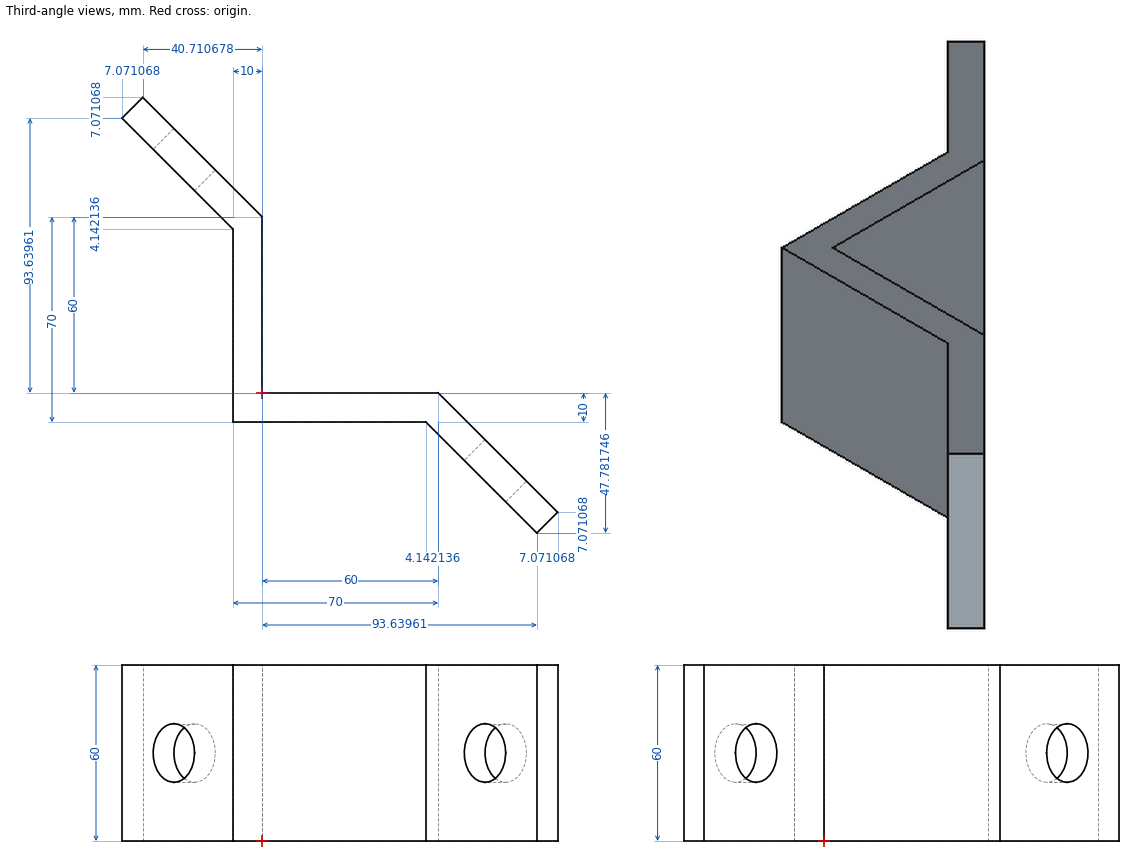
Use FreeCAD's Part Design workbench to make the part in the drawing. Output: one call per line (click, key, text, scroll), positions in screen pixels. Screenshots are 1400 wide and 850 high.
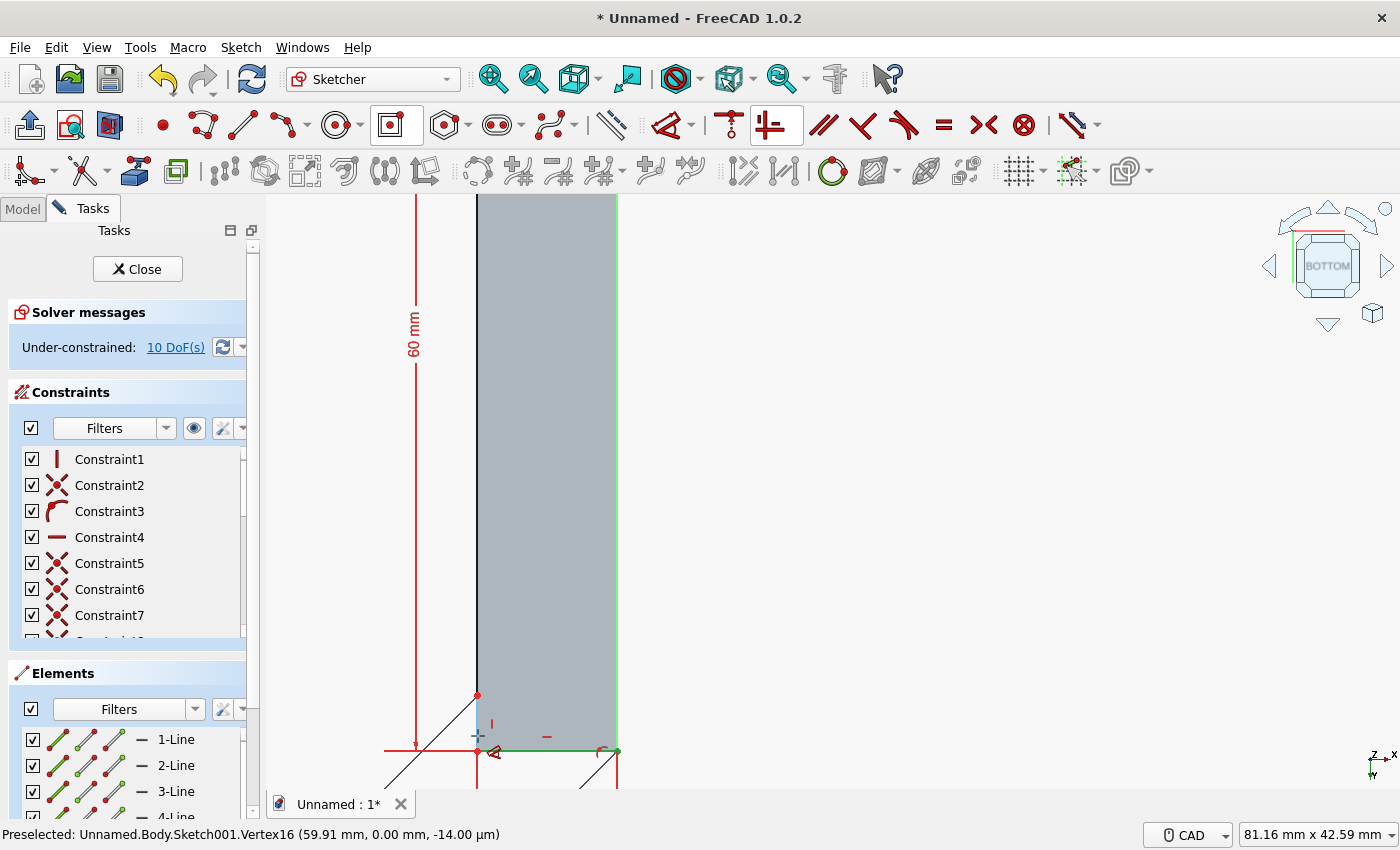
click(477, 735)
click(443, 711)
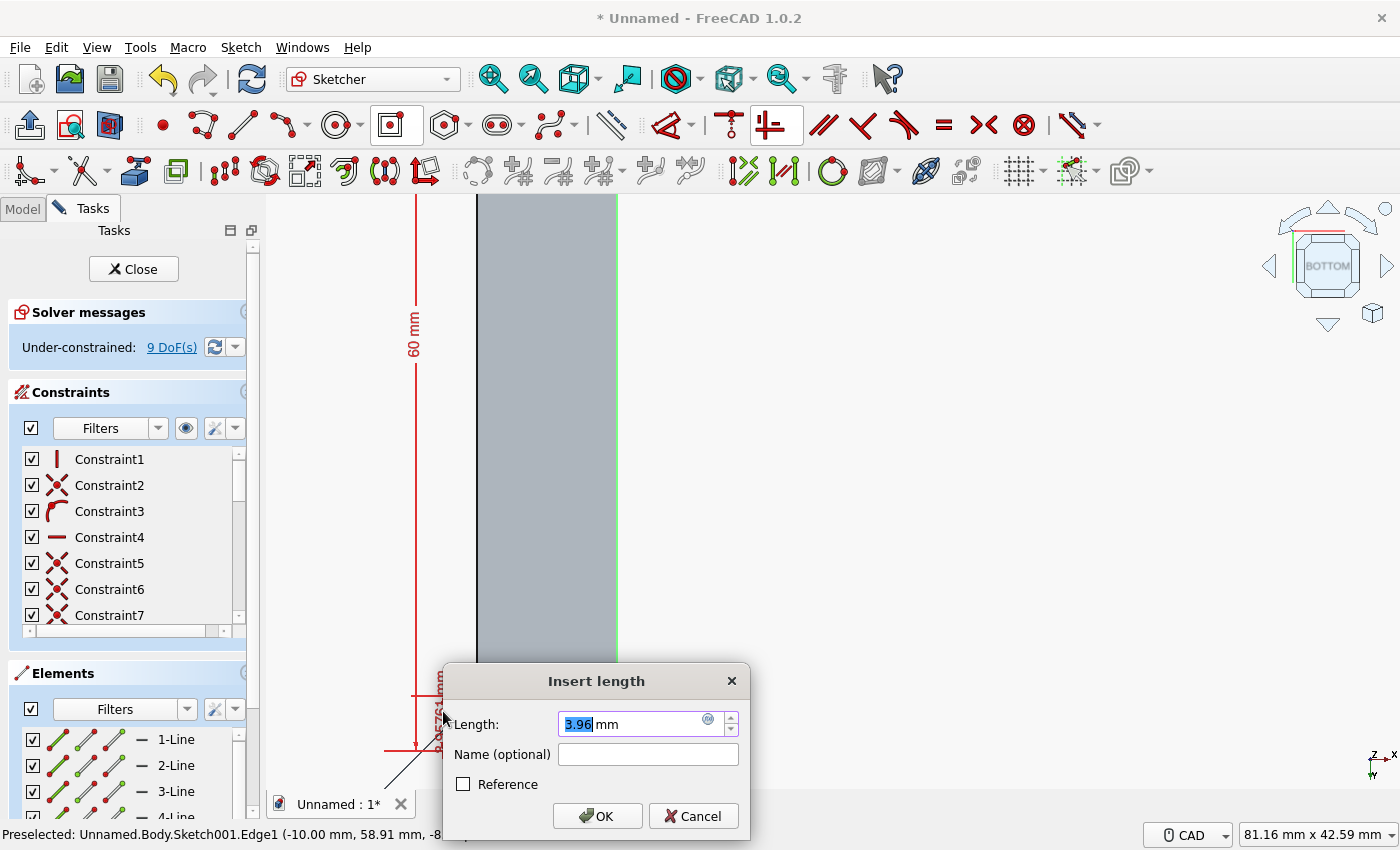
text(4.142136)
key(Return)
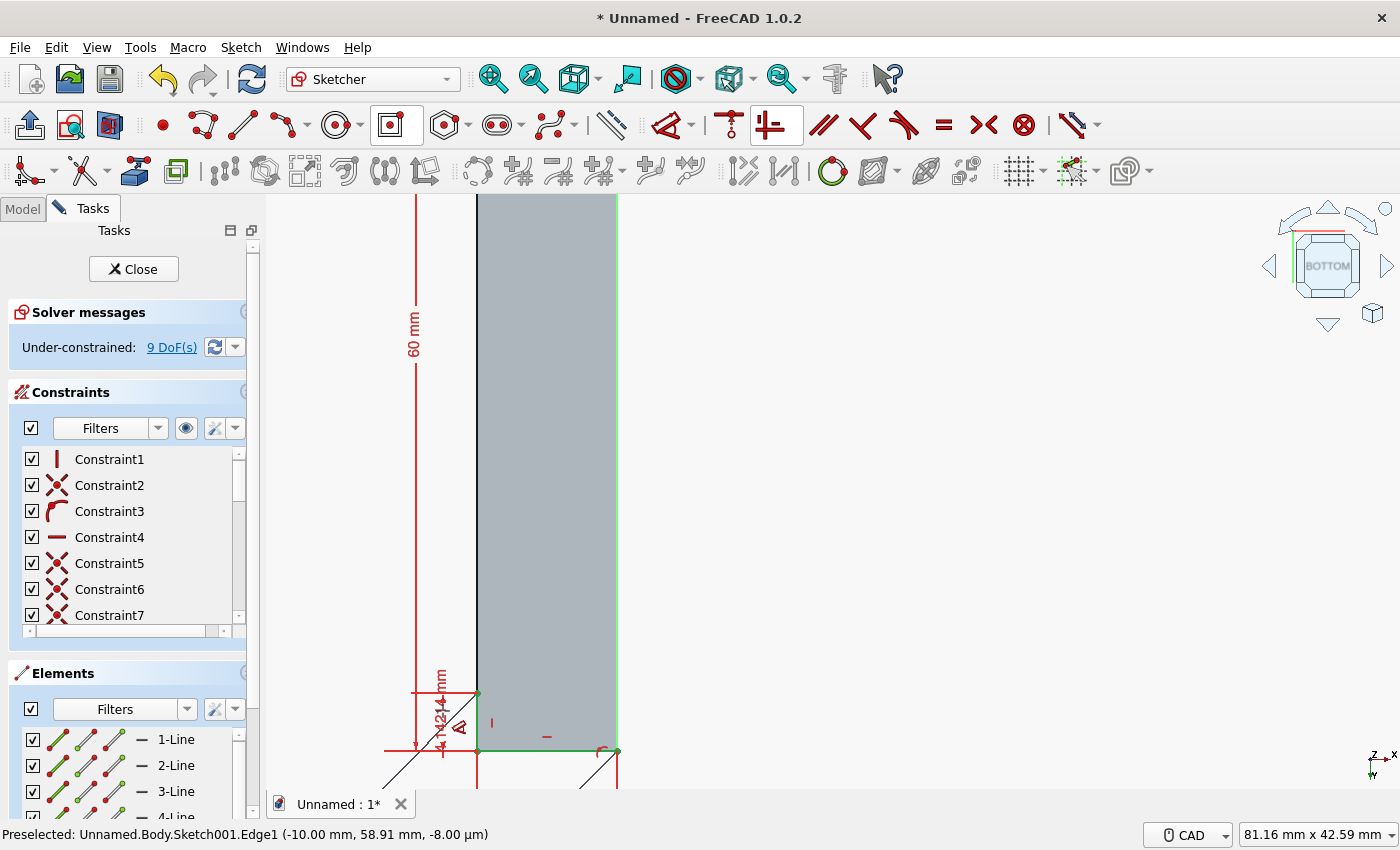
scroll(708, 544, down, 8)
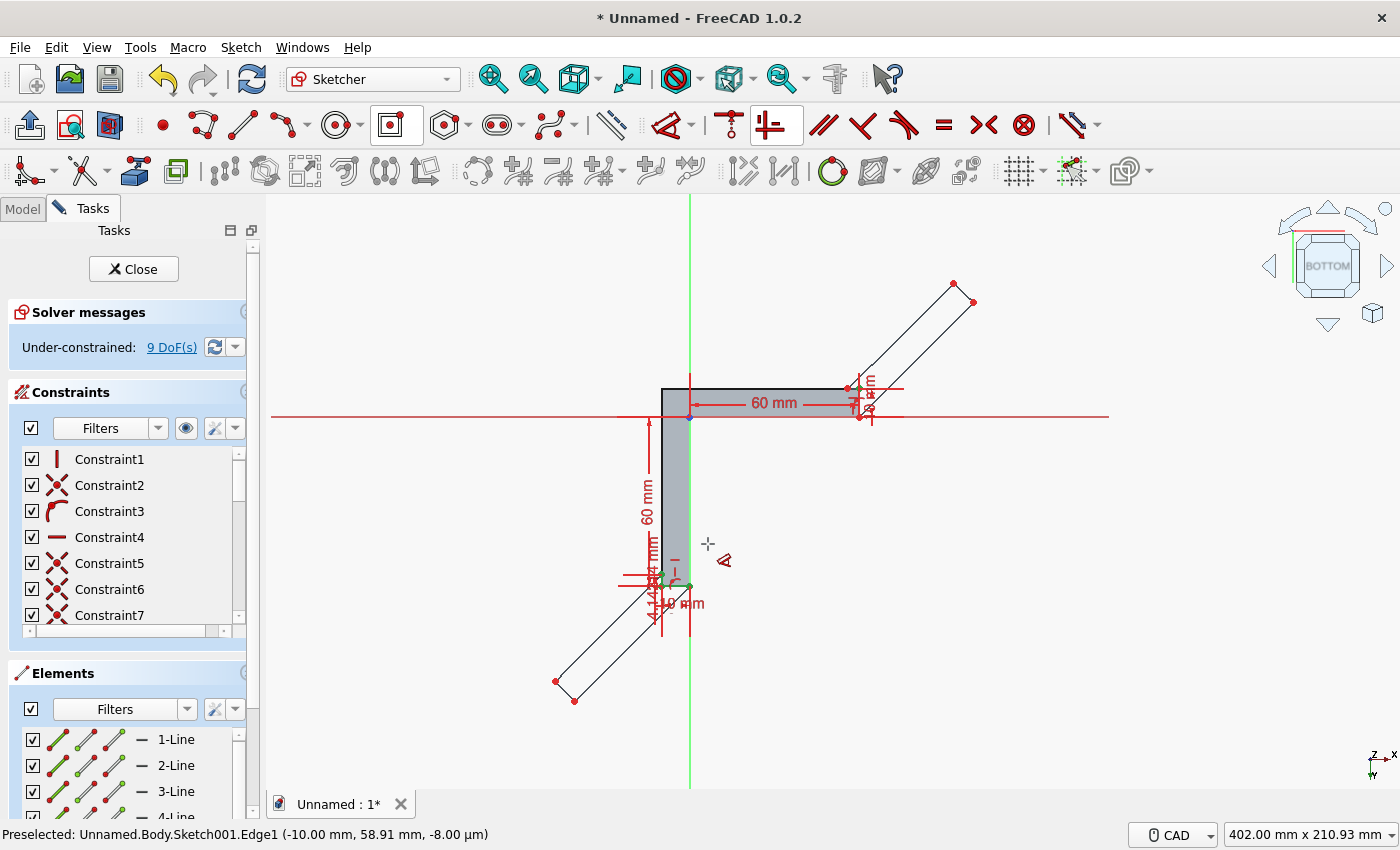
scroll(856, 389, up, 8)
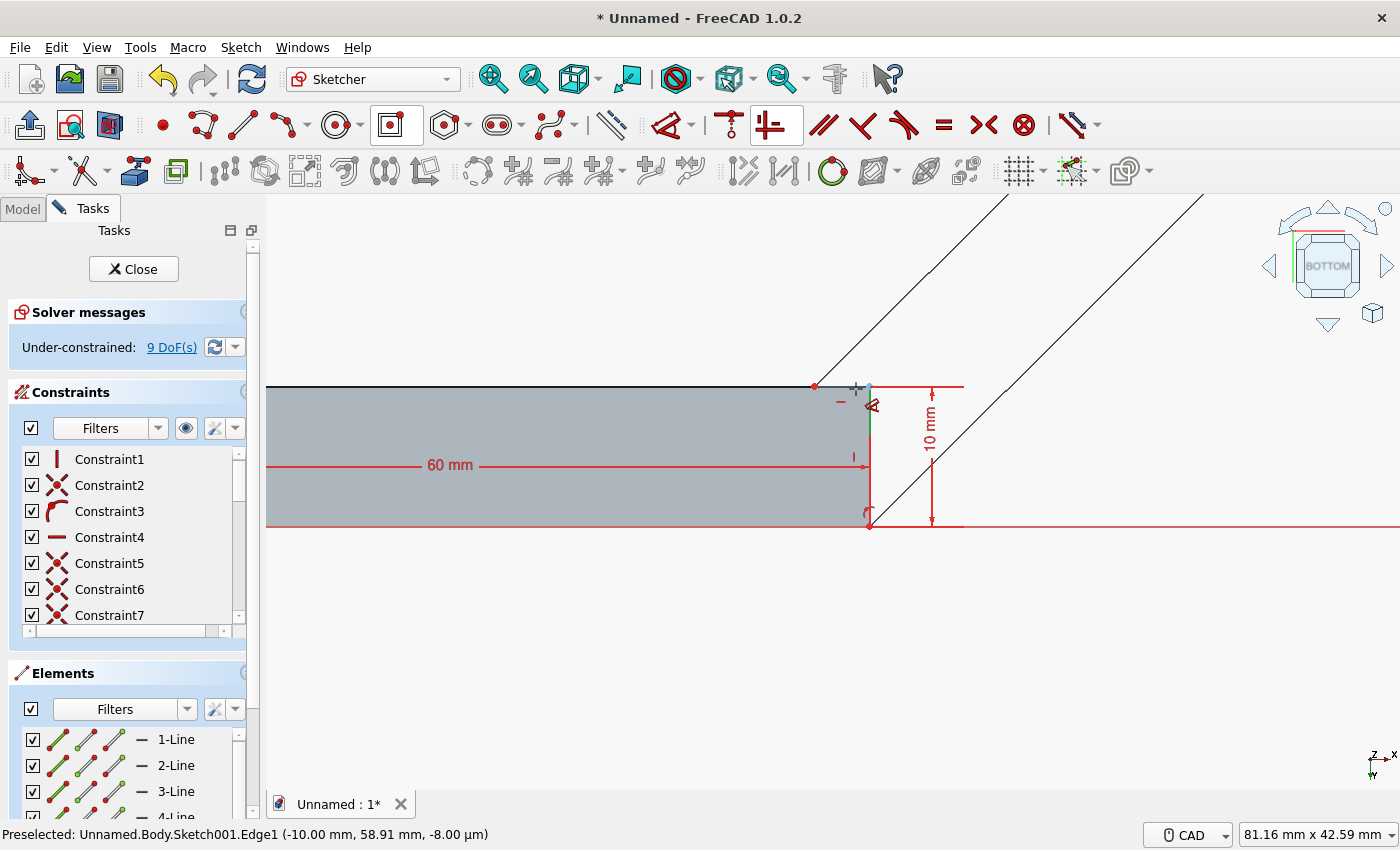
click(853, 387)
click(829, 353)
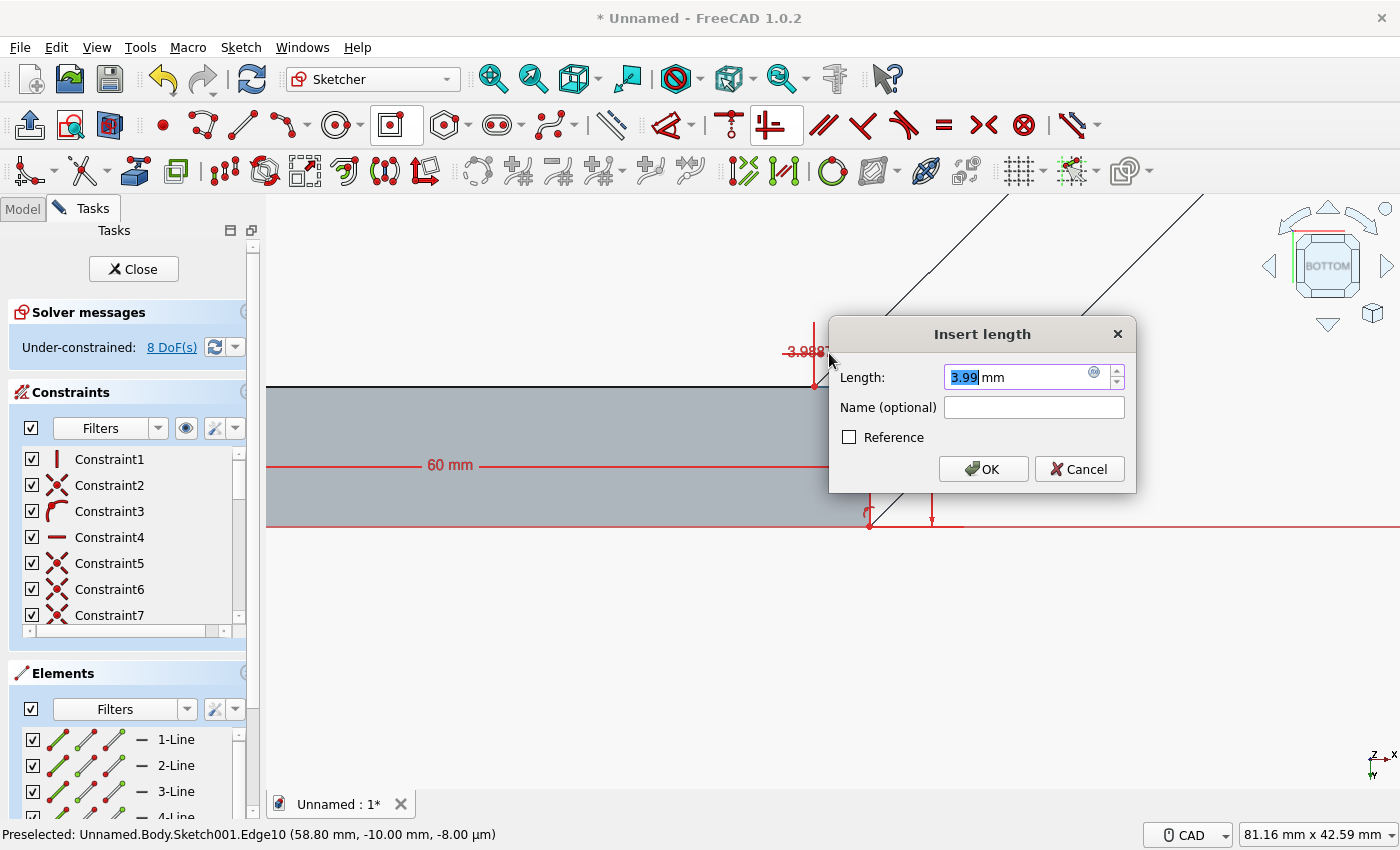
text(4.142136)
key(Return)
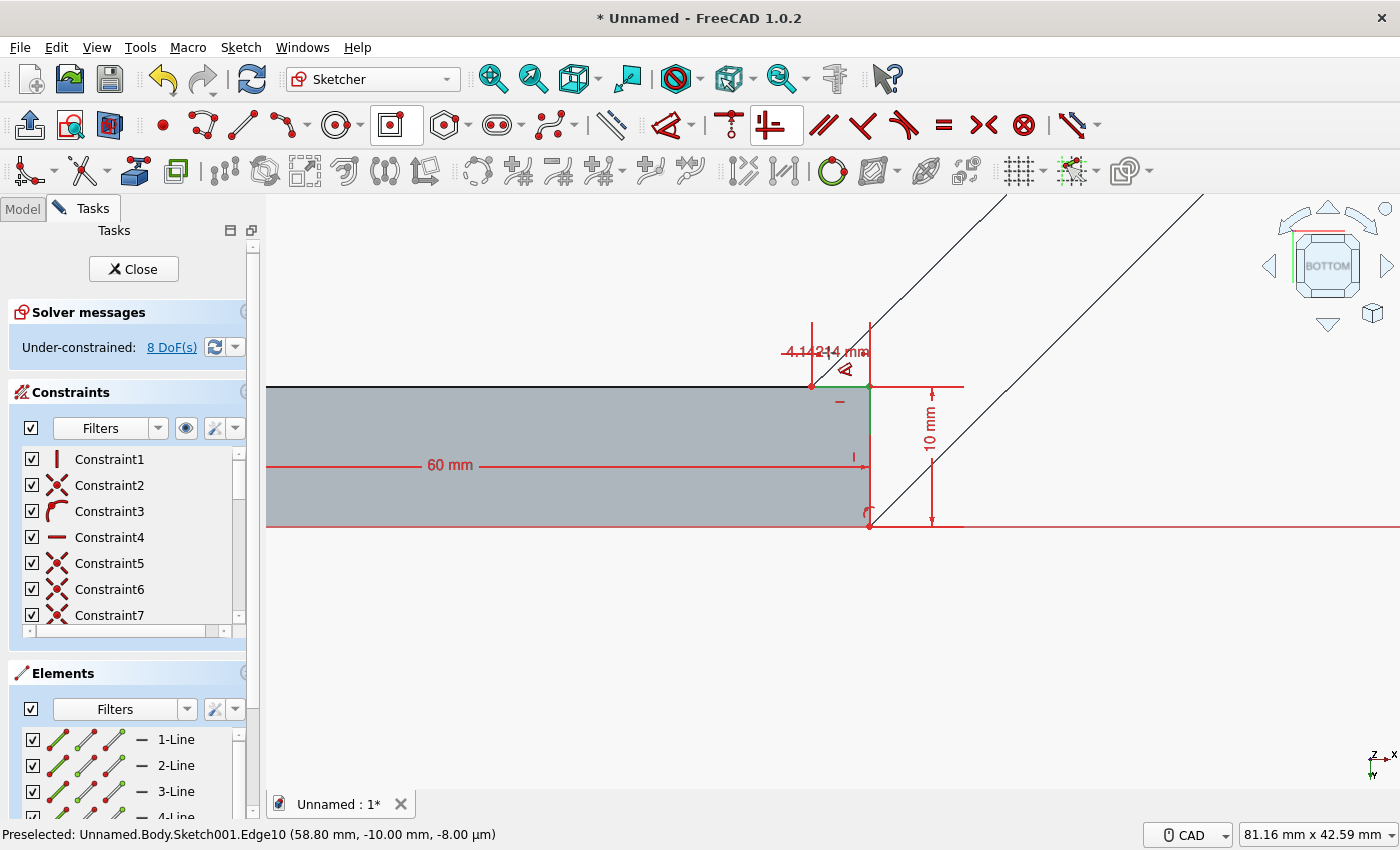
scroll(856, 389, down, 8)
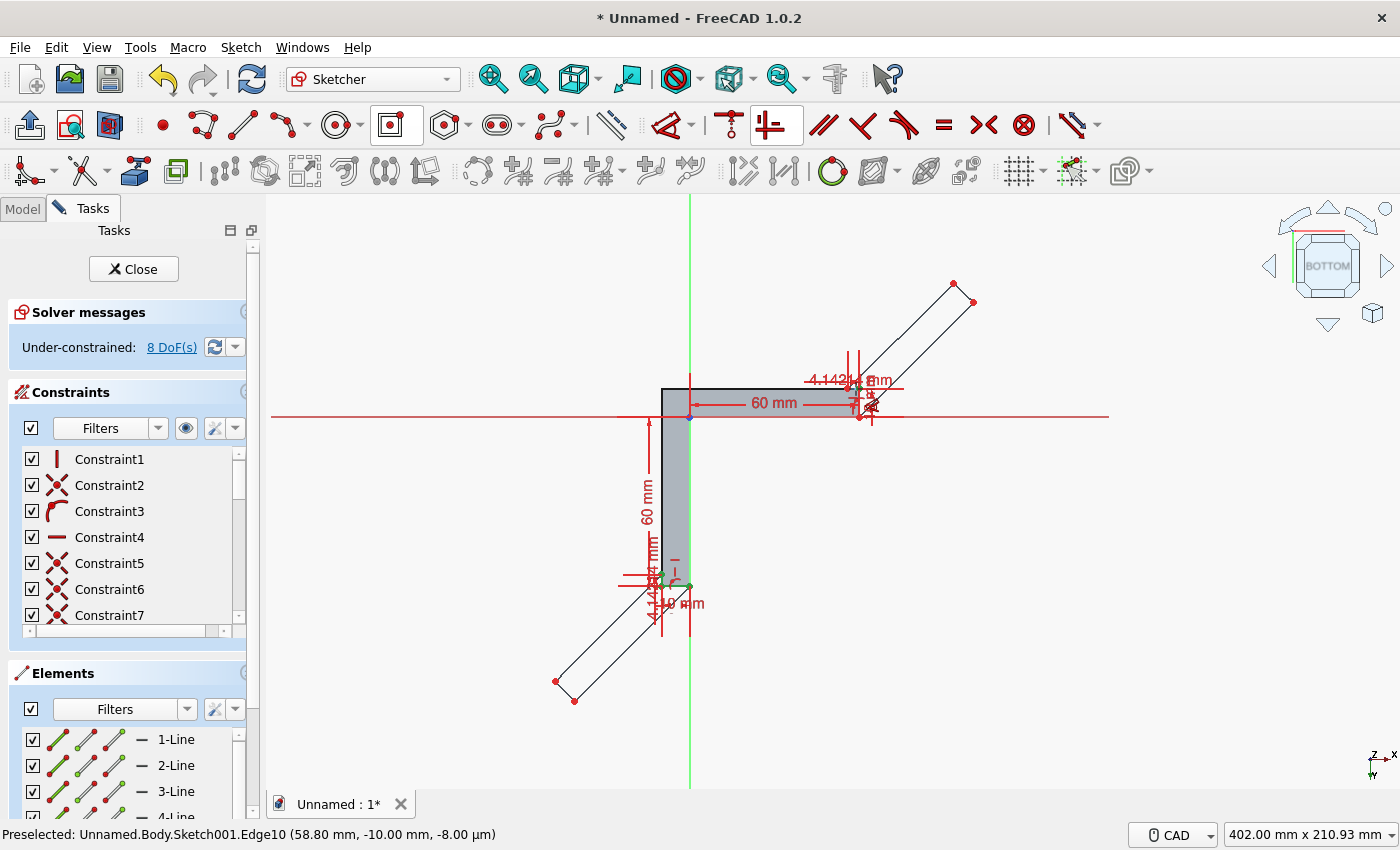
click(555, 682)
click(521, 549)